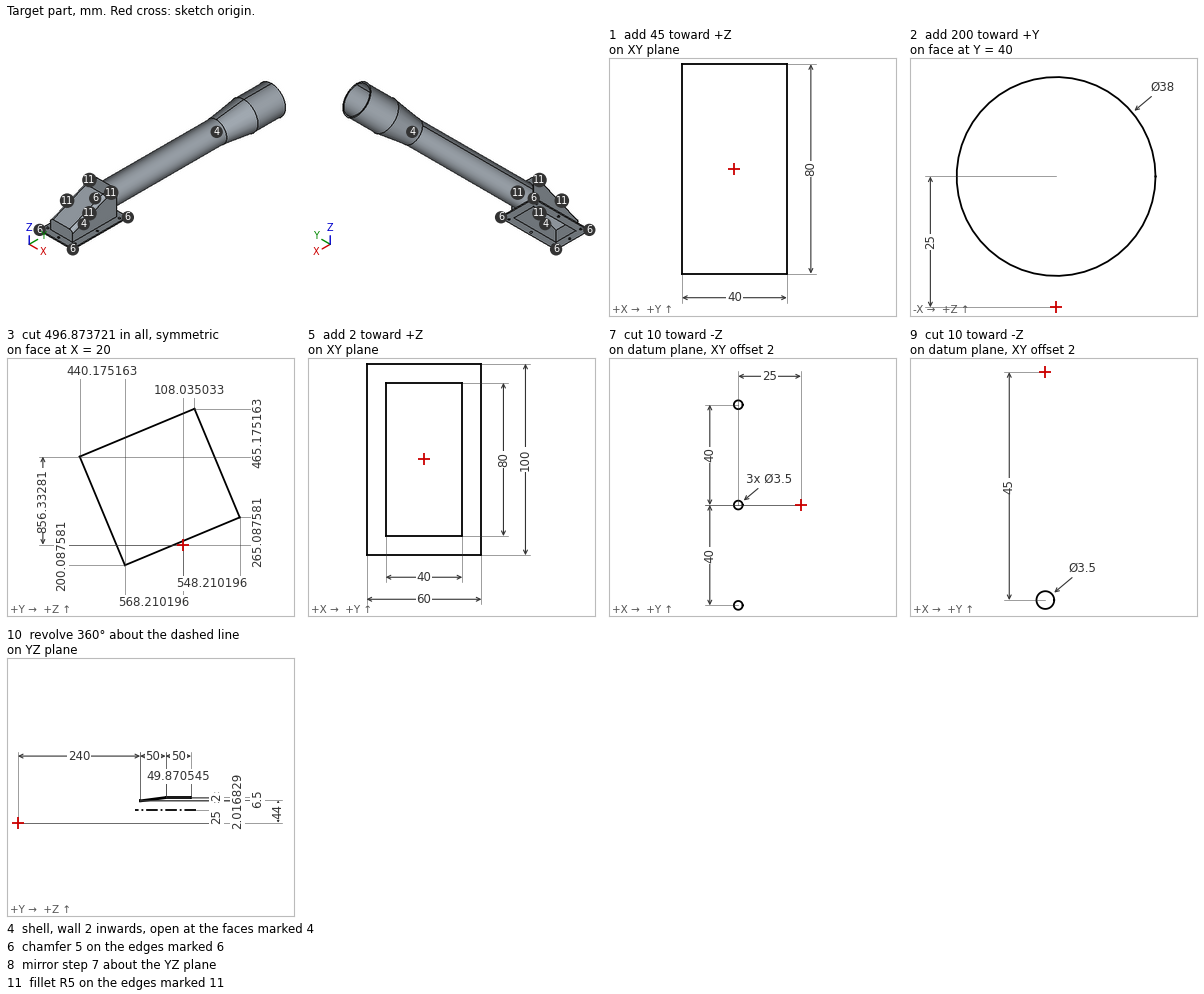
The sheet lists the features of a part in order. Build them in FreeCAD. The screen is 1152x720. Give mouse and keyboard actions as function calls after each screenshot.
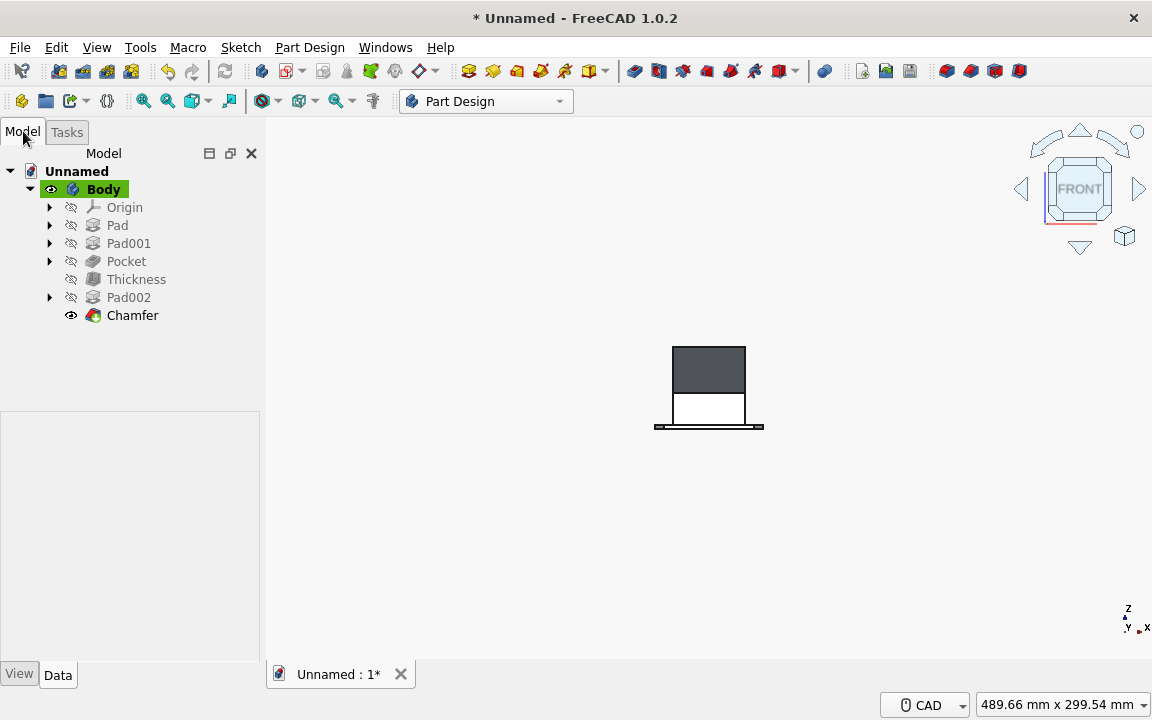
click(50, 207)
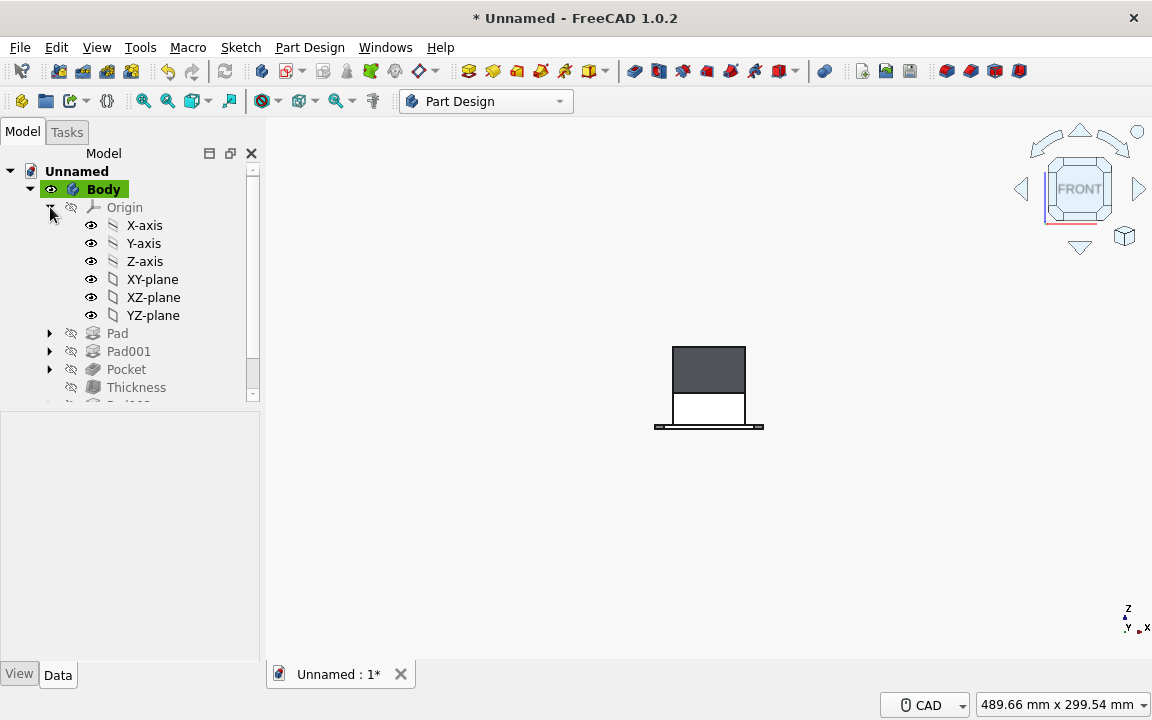
click(136, 279)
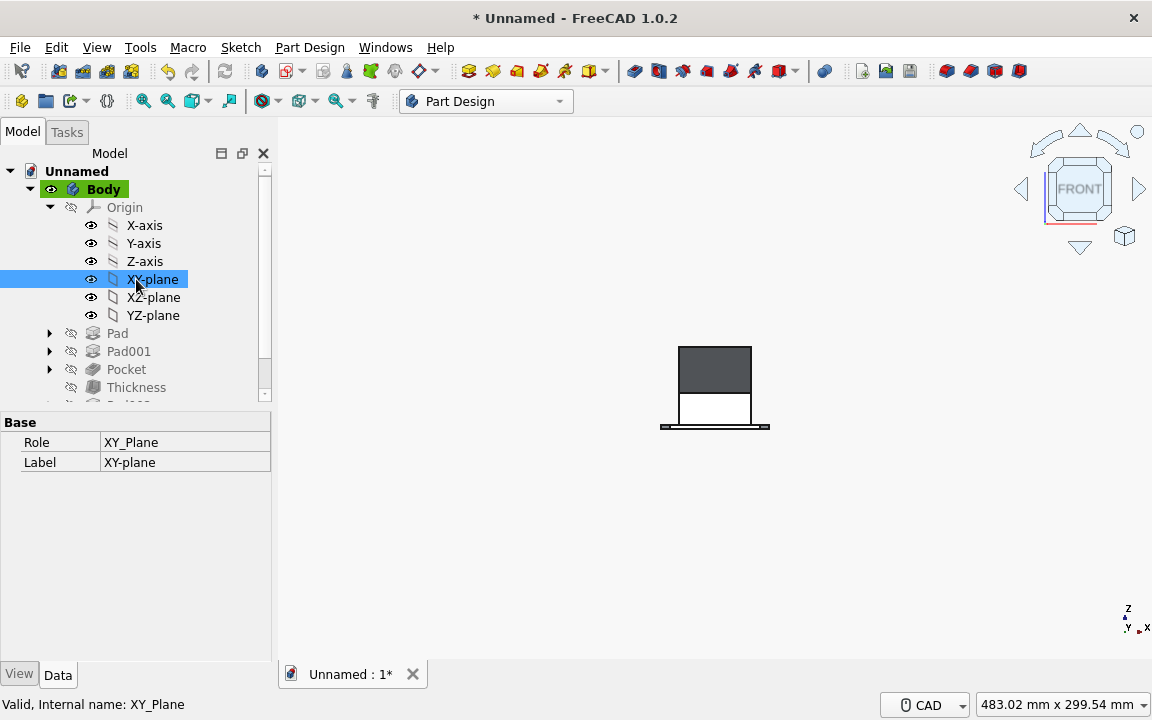
click(420, 72)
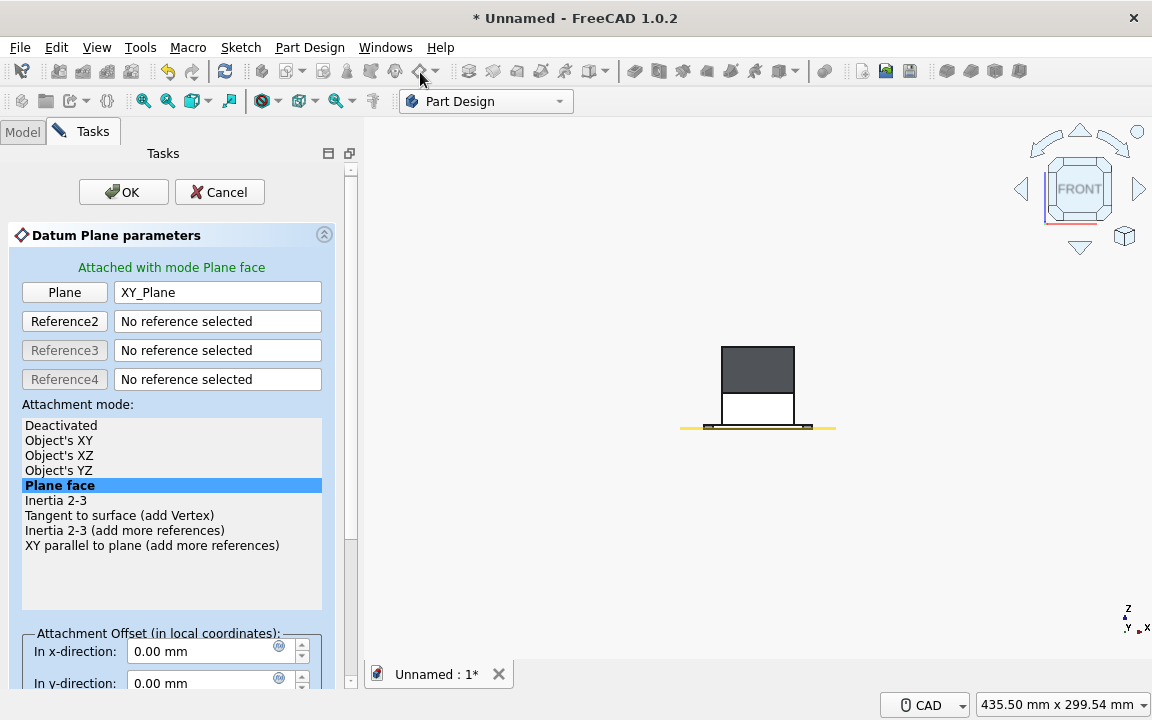
scroll(351, 426, down, 2)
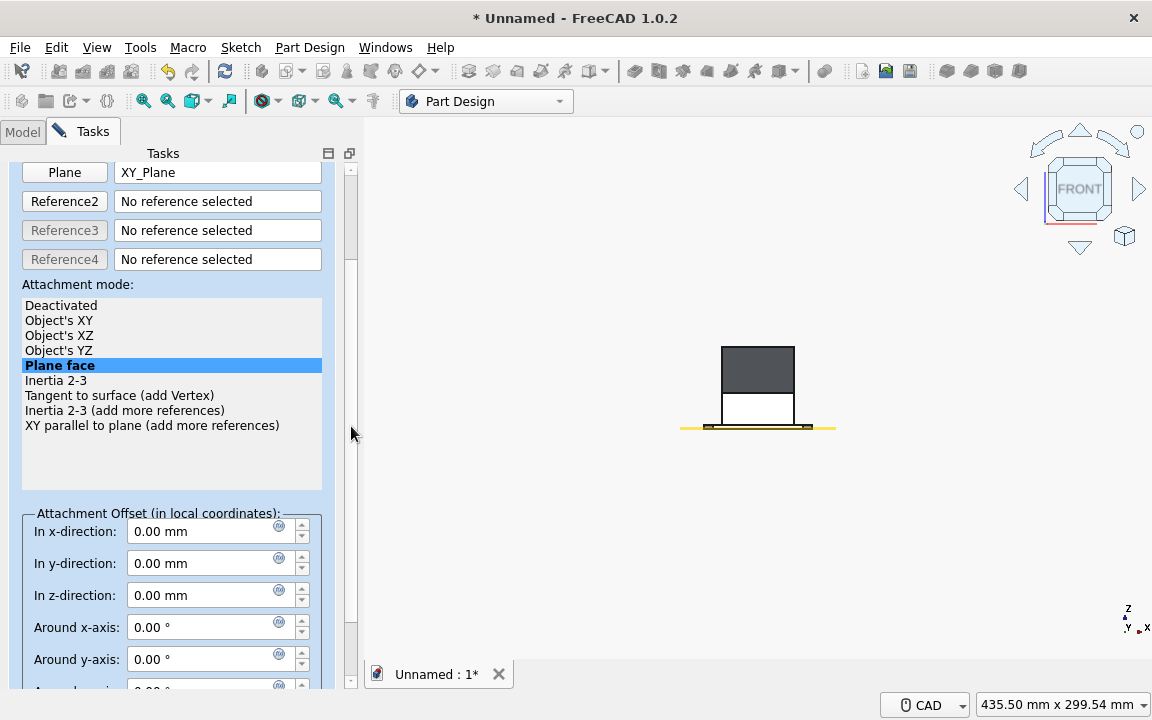
triple_click(210, 595)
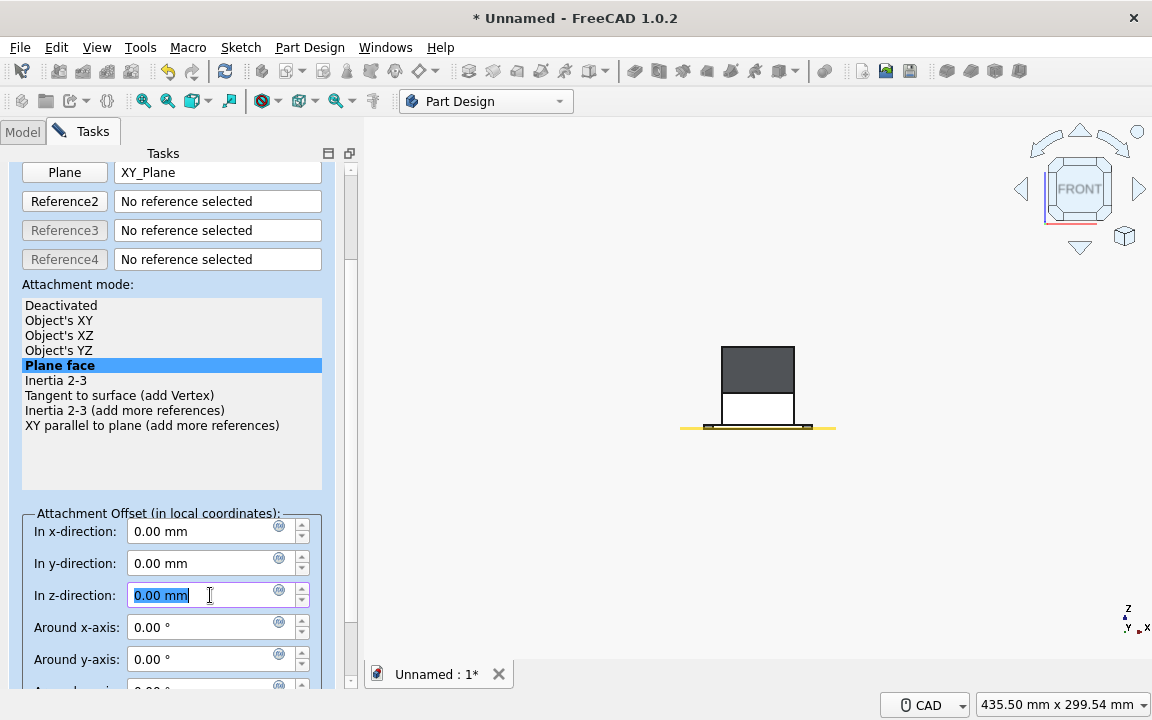
text(2)
key(Tab)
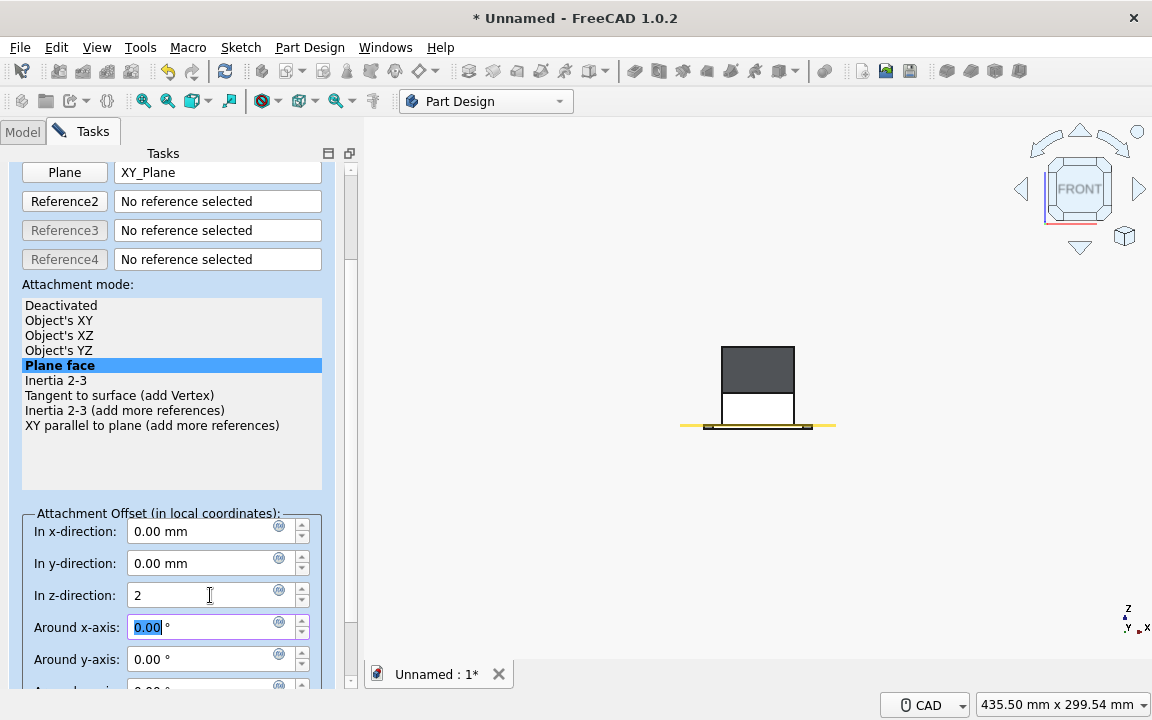
scroll(351, 426, up, 3)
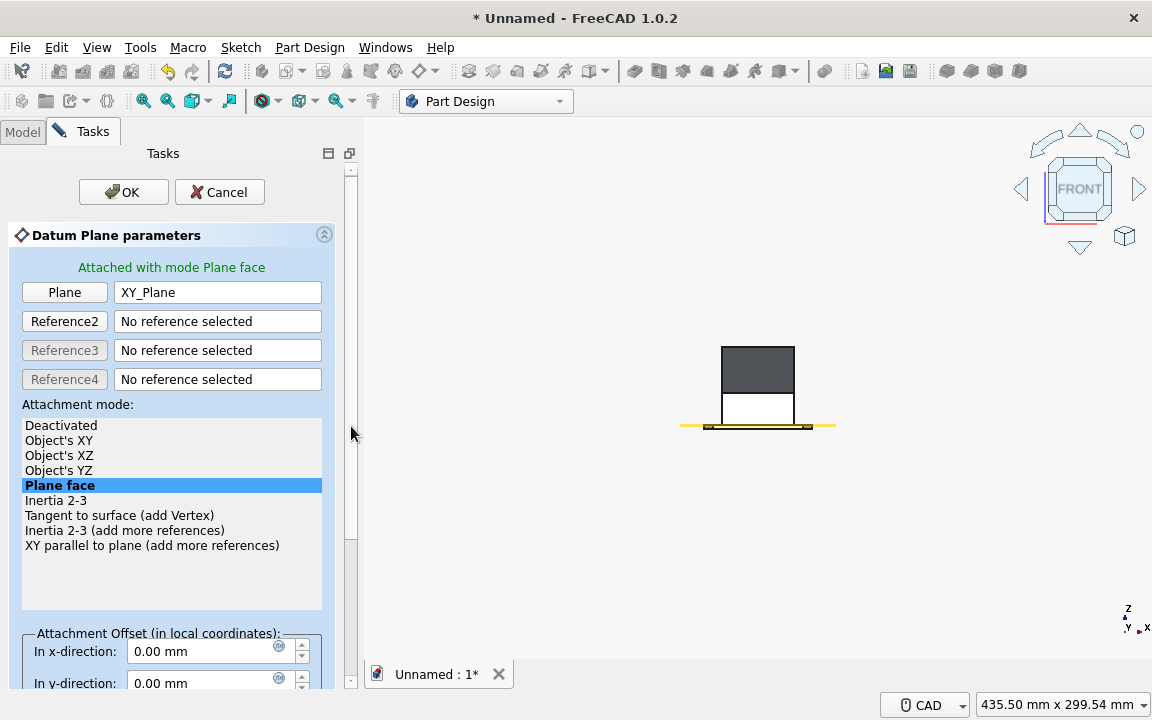
click(124, 192)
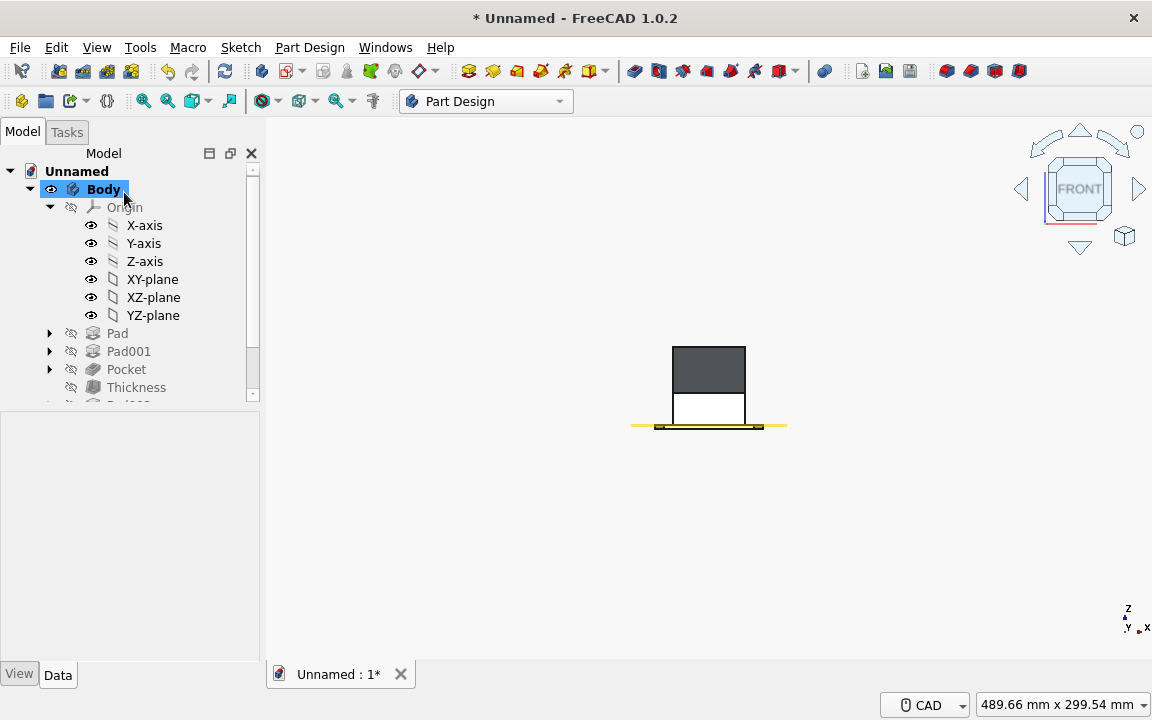
scroll(100, 275, down, 3)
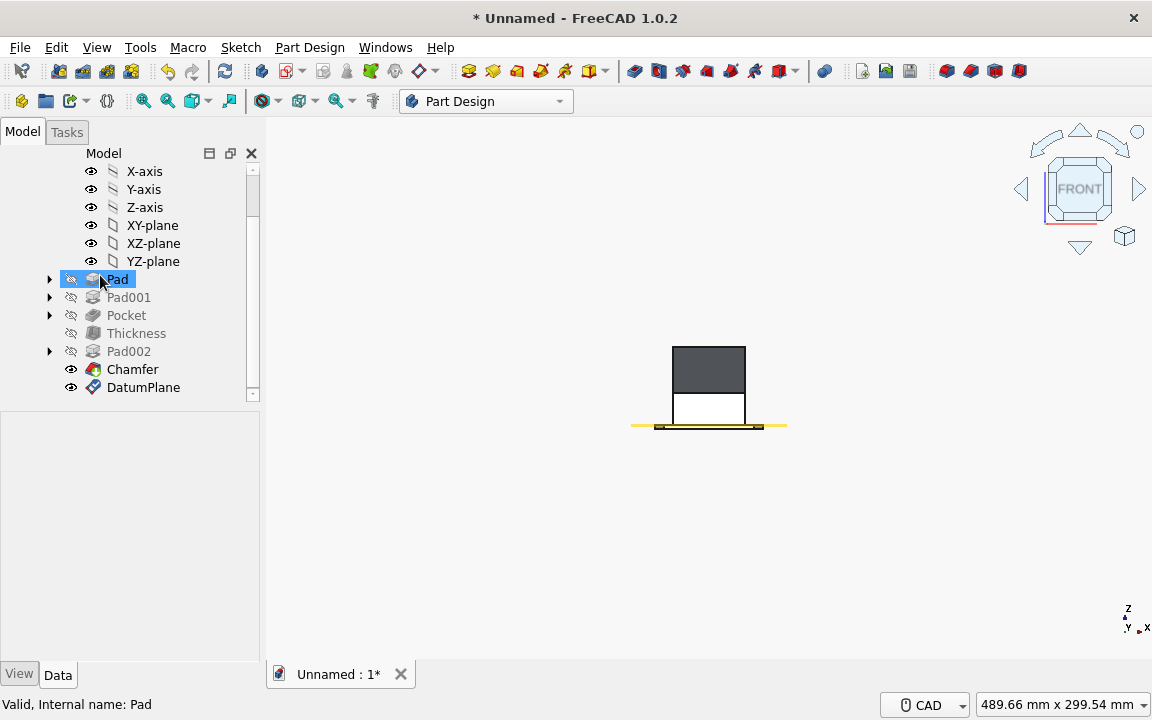
click(116, 387)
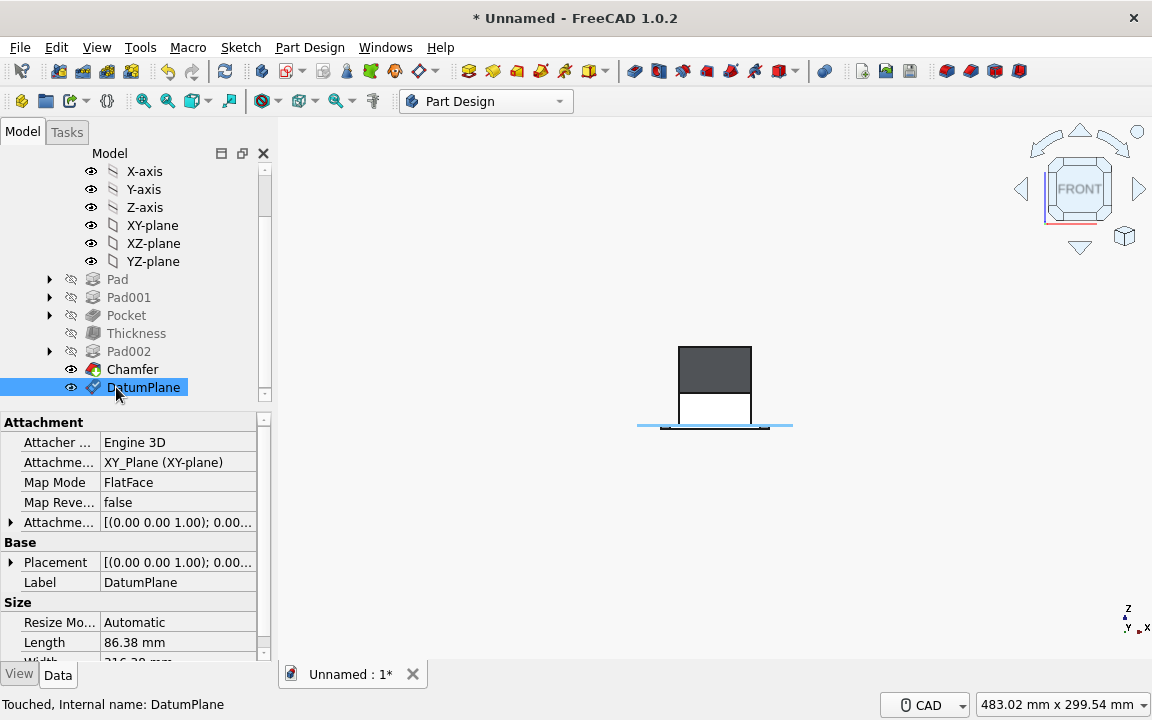
click(286, 72)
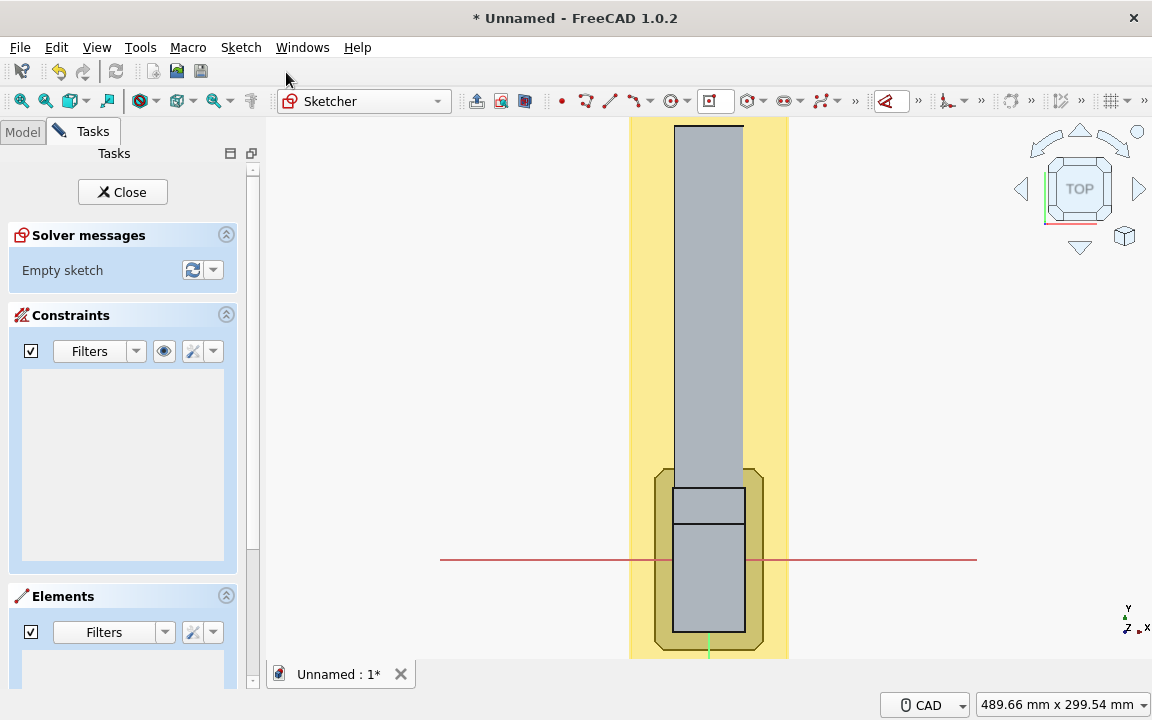
key(q)
key(s)